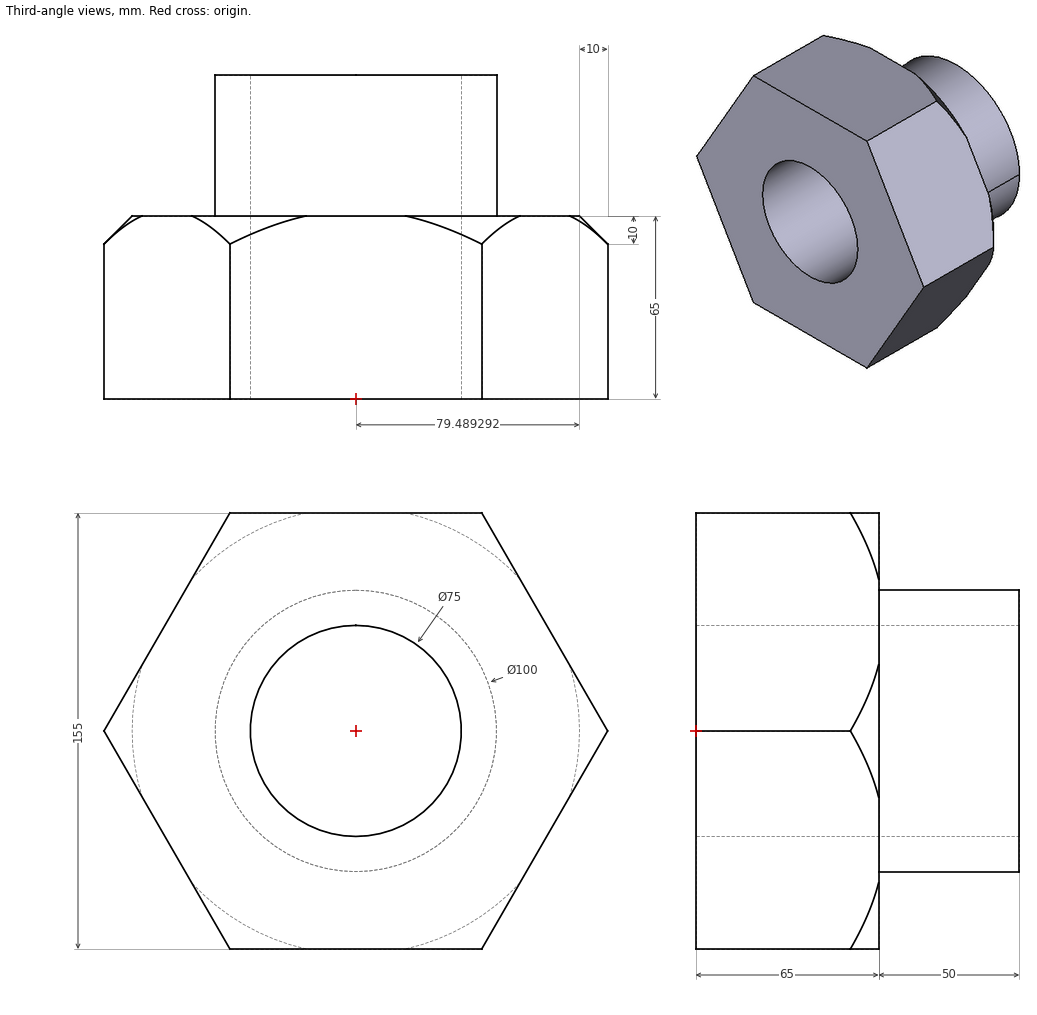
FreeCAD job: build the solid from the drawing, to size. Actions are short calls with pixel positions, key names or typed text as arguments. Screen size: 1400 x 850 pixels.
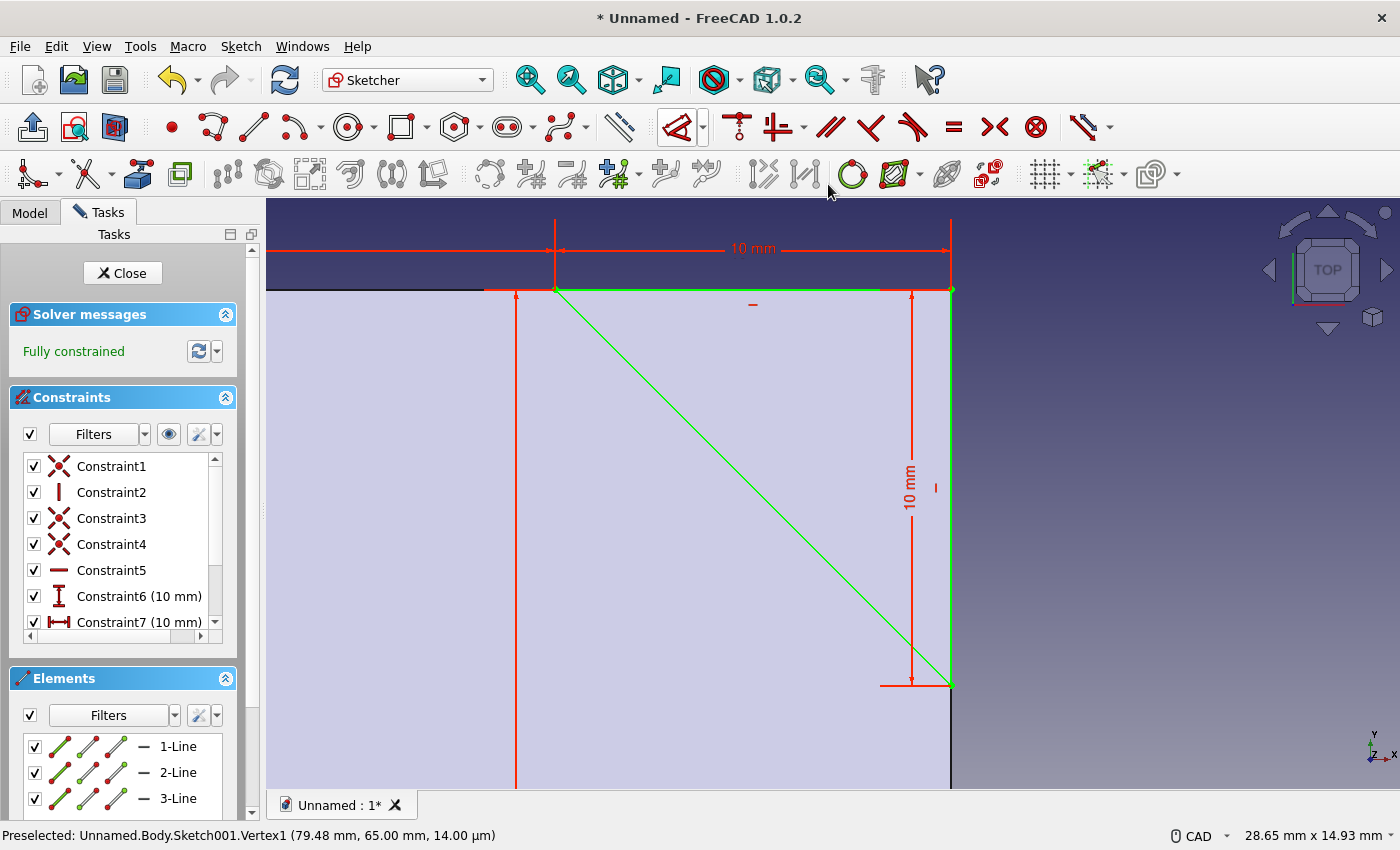
click(123, 273)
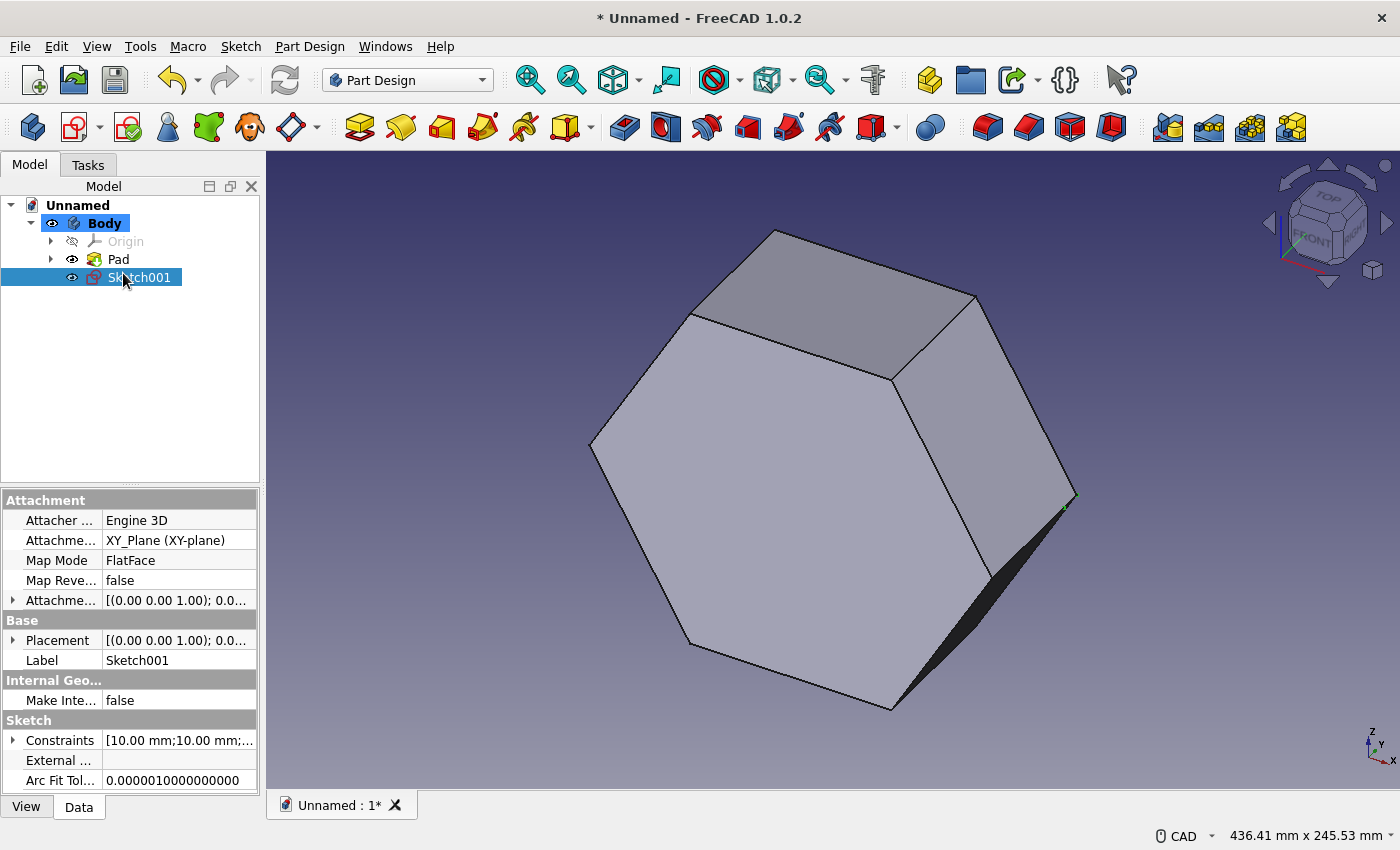
click(707, 128)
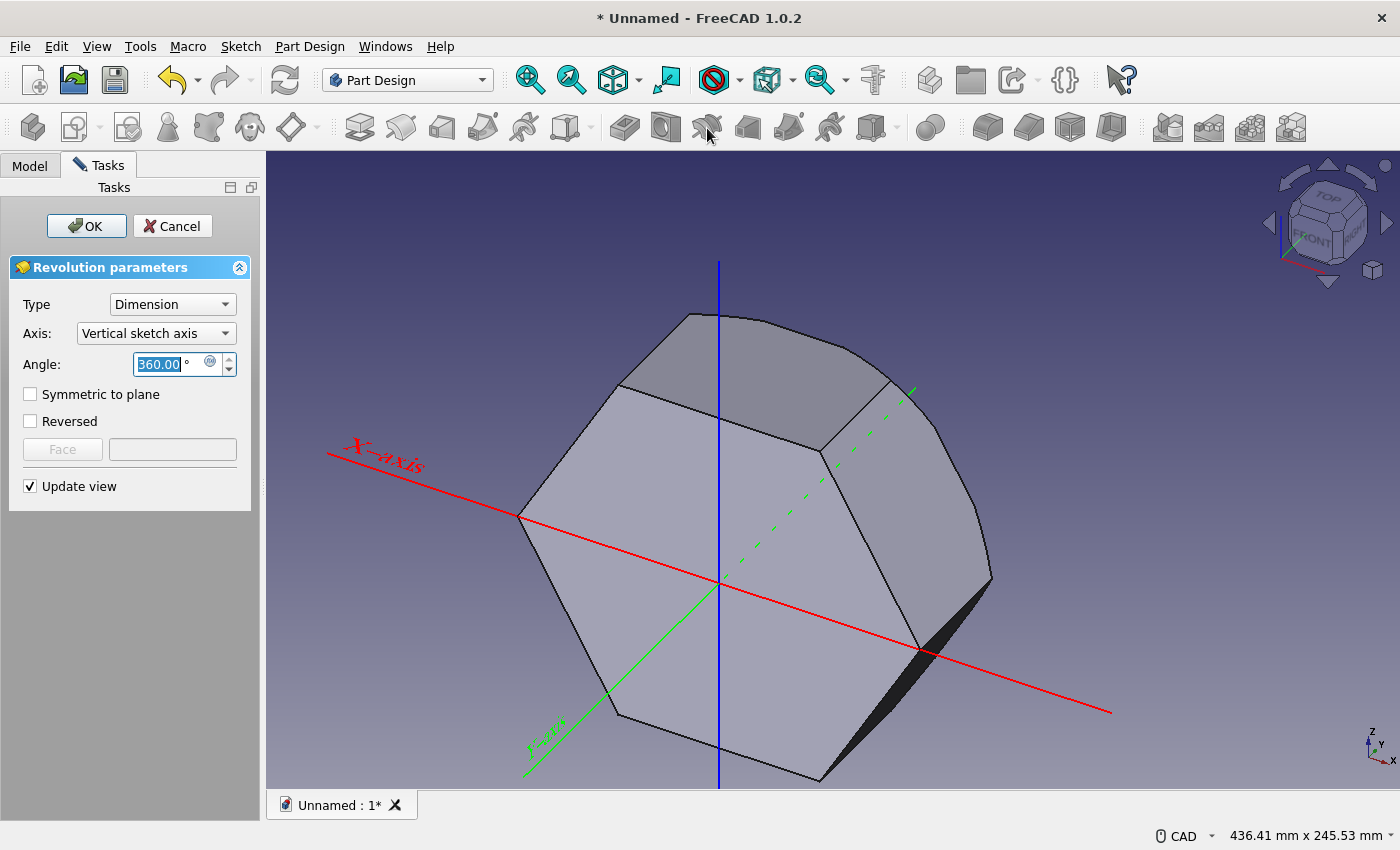
click(87, 226)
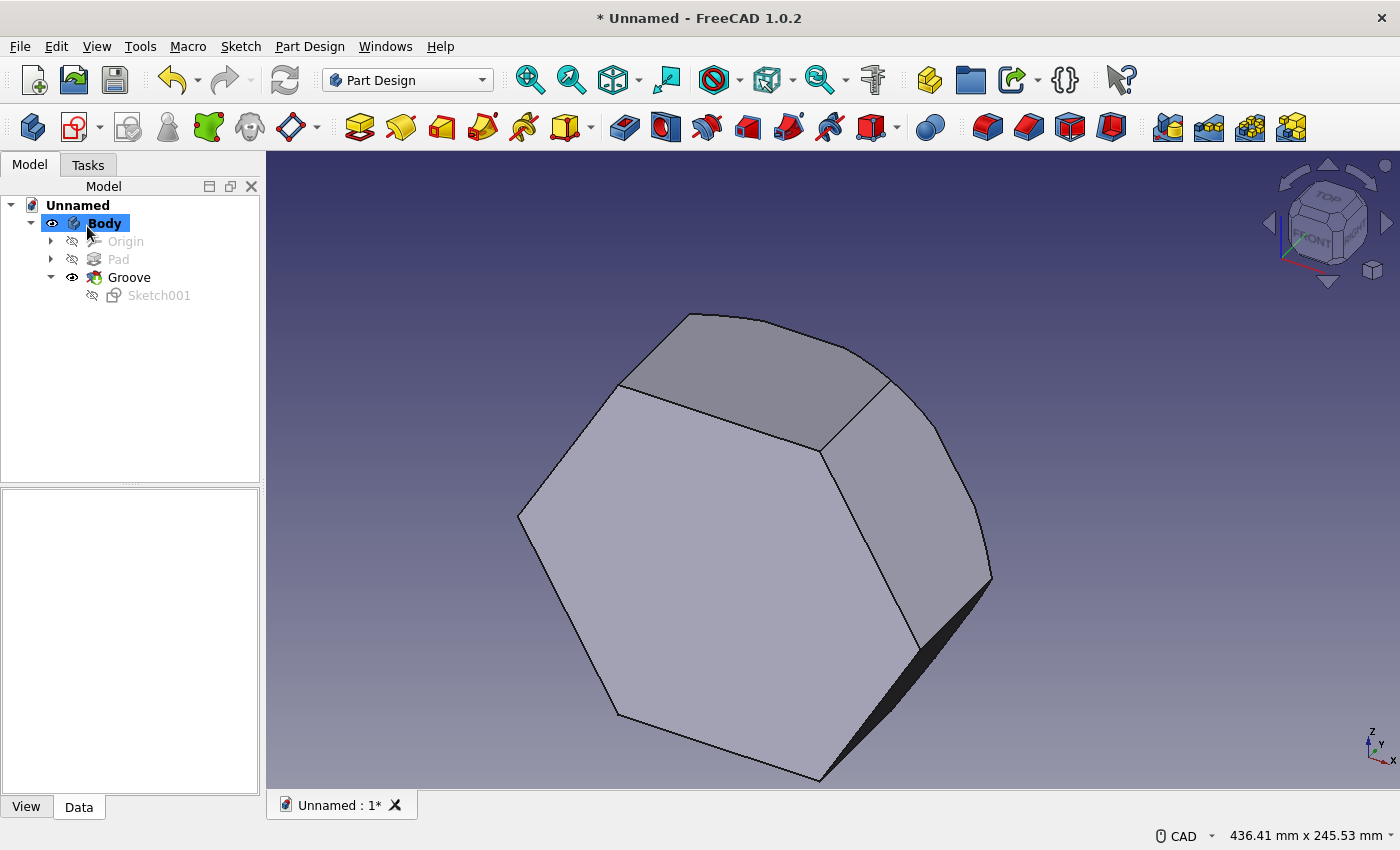
click(531, 80)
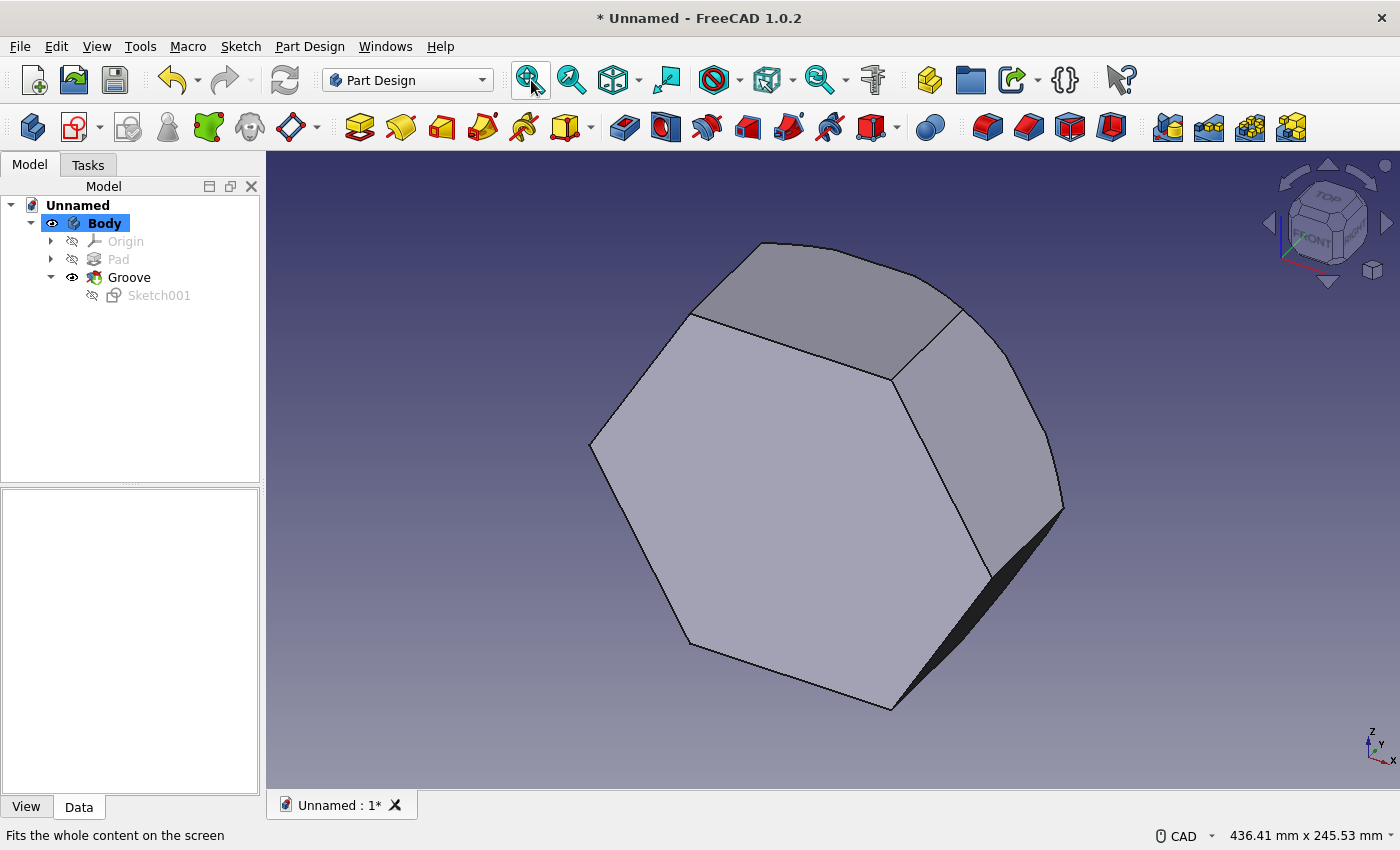
key(4)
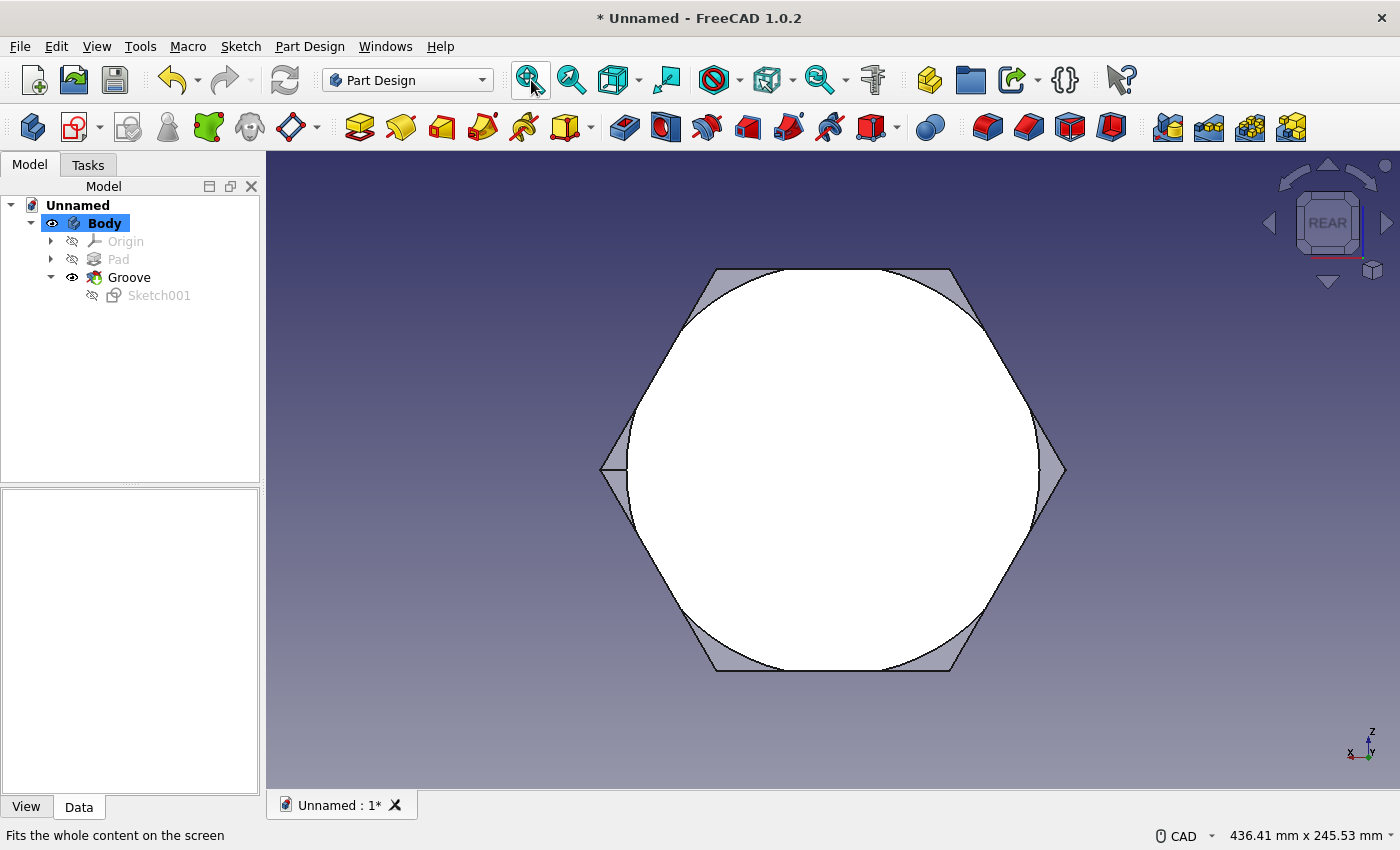
click(833, 469)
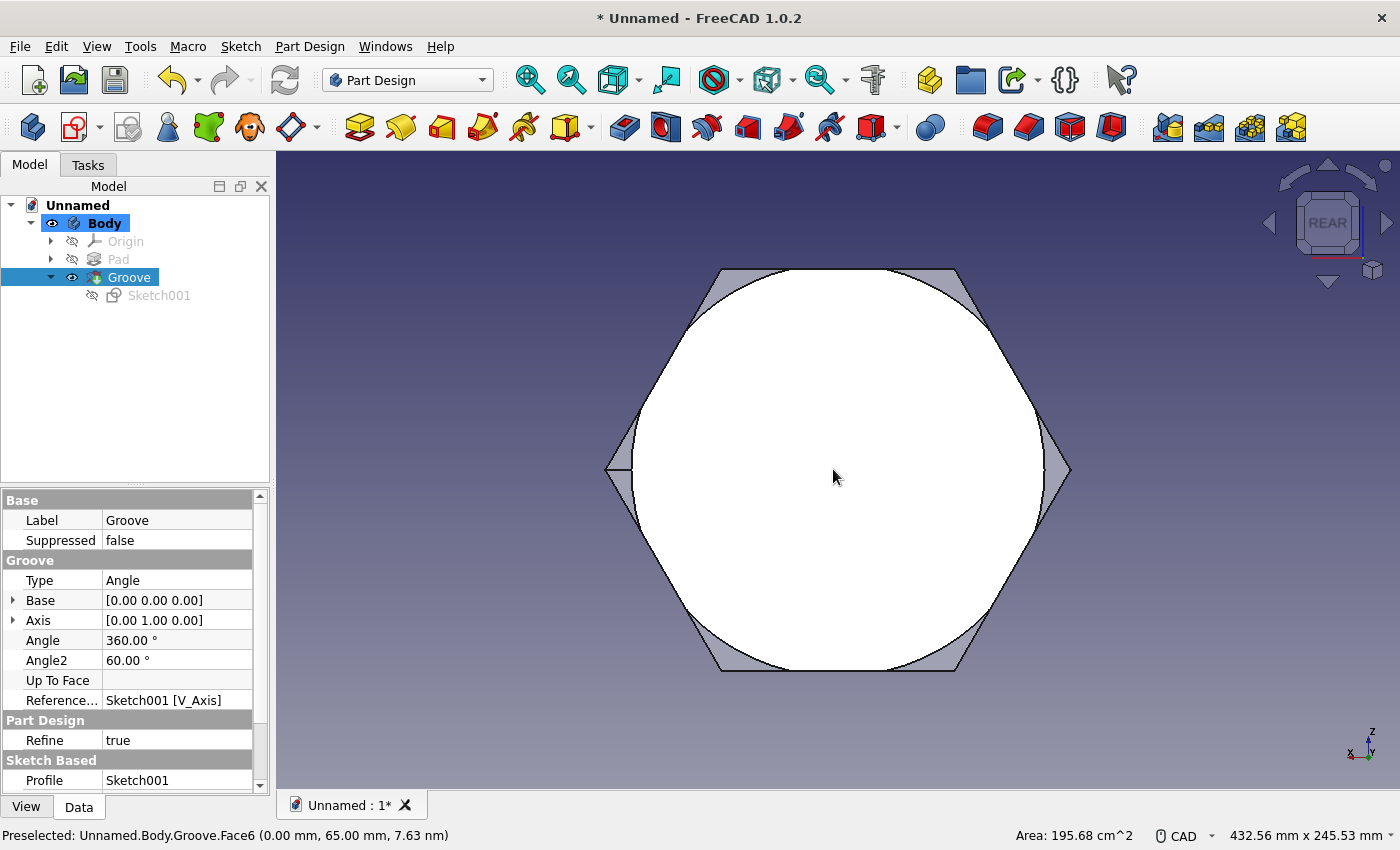
click(74, 128)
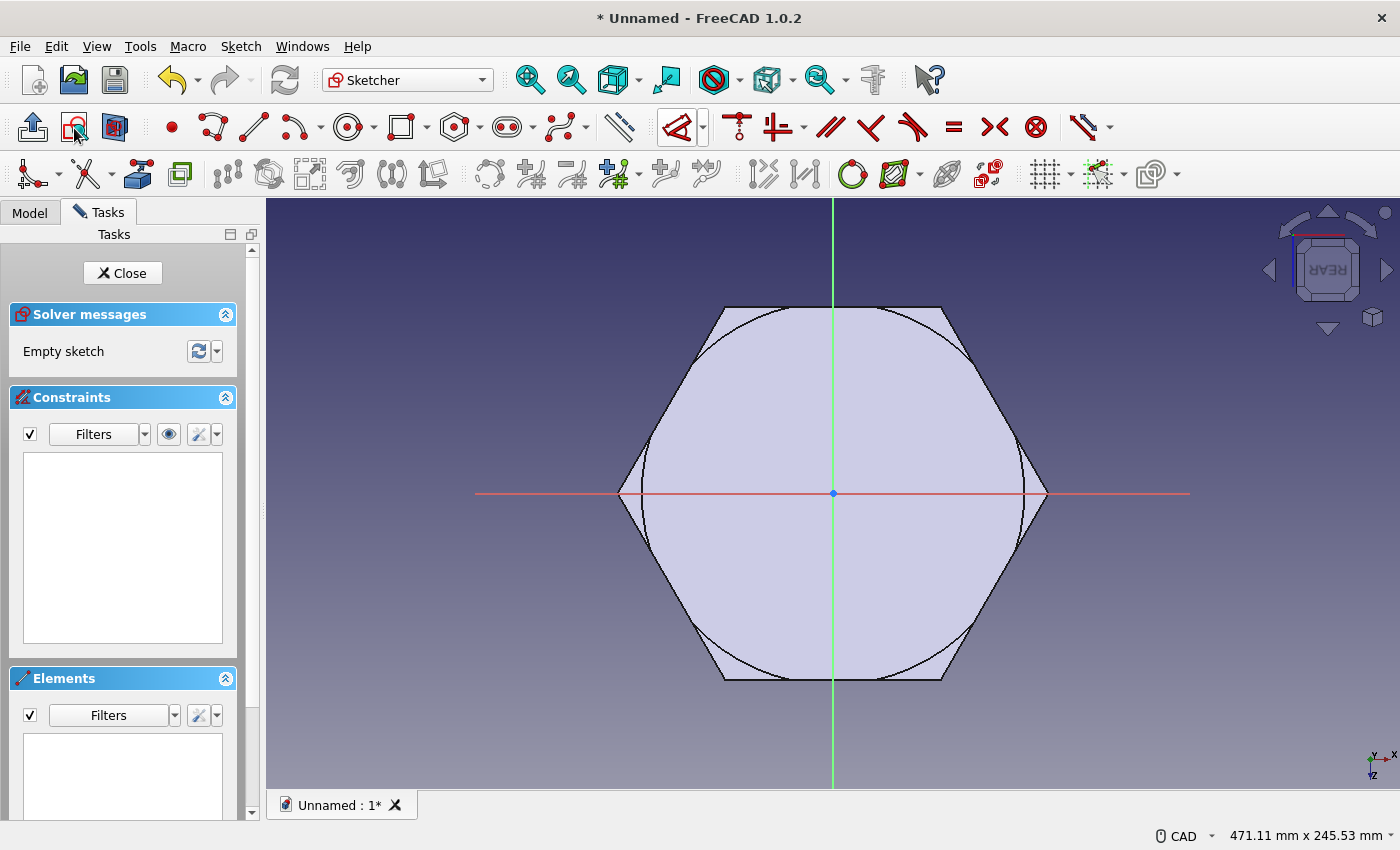
scroll(972, 493, up, 2)